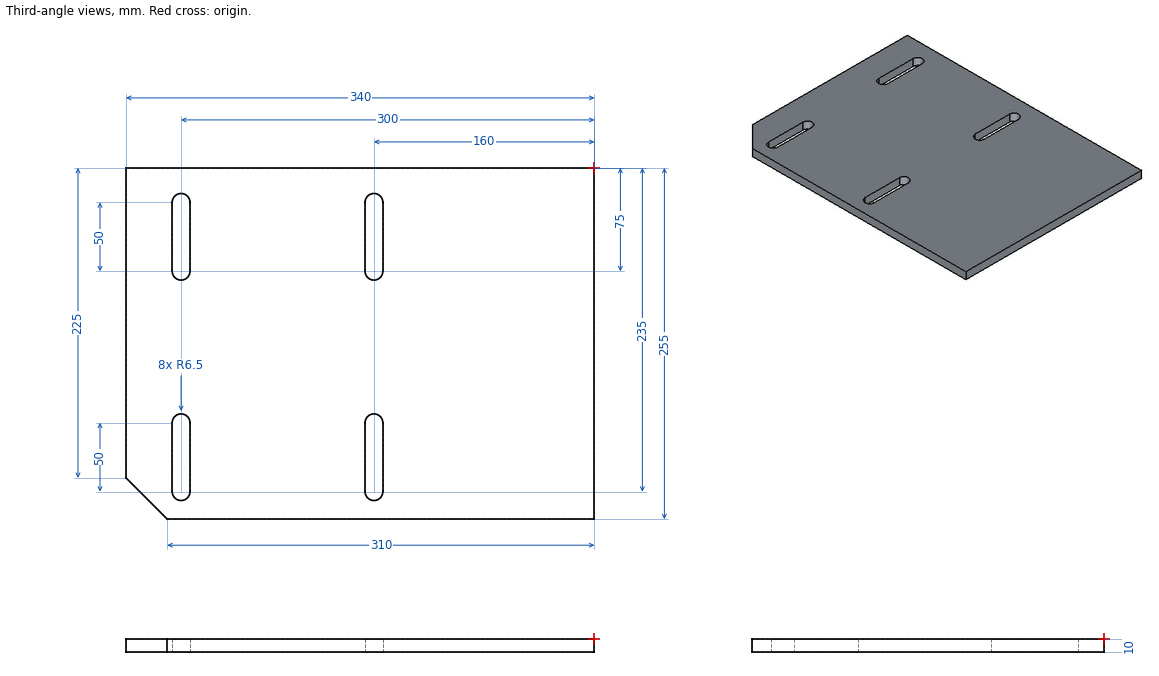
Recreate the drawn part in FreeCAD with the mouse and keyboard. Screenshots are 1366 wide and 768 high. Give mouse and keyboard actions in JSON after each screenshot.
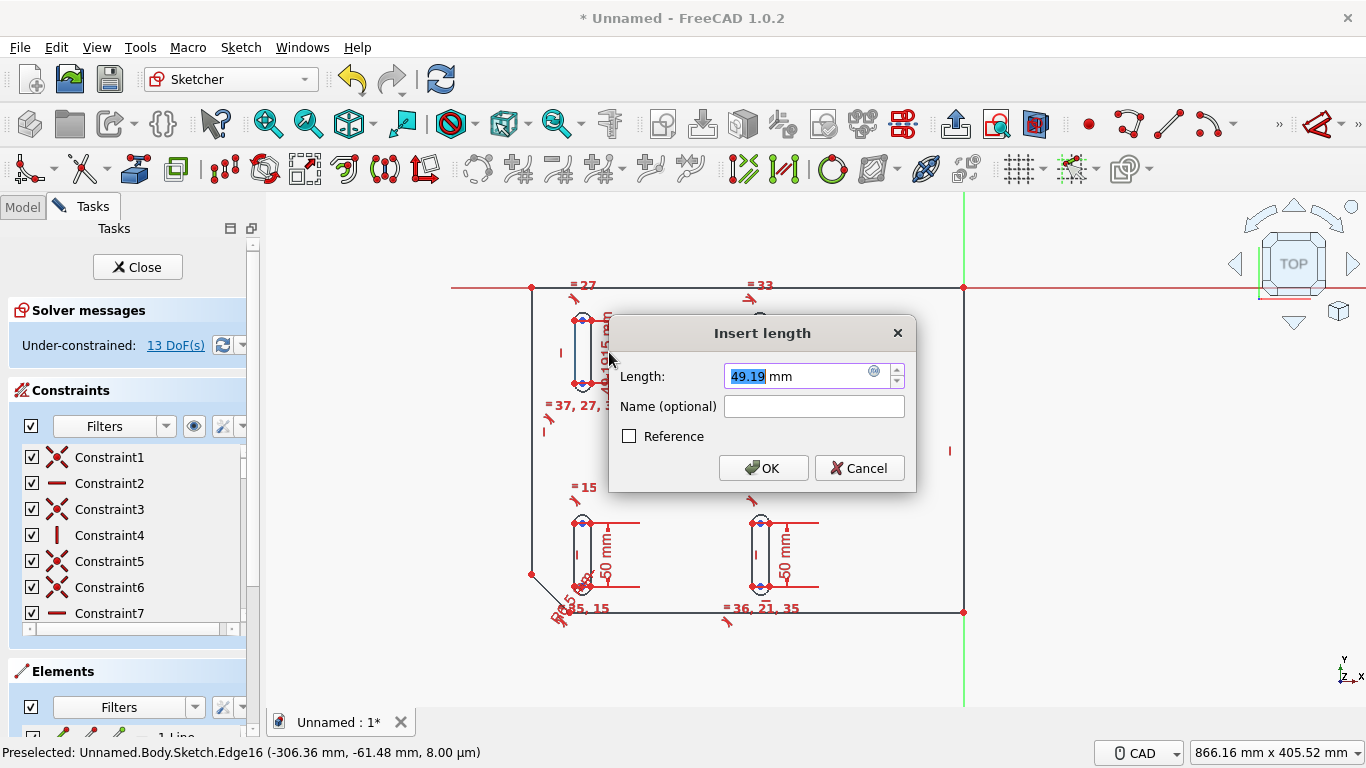
{"action": "type", "text": "50"}
{"action": "key", "text": "Return"}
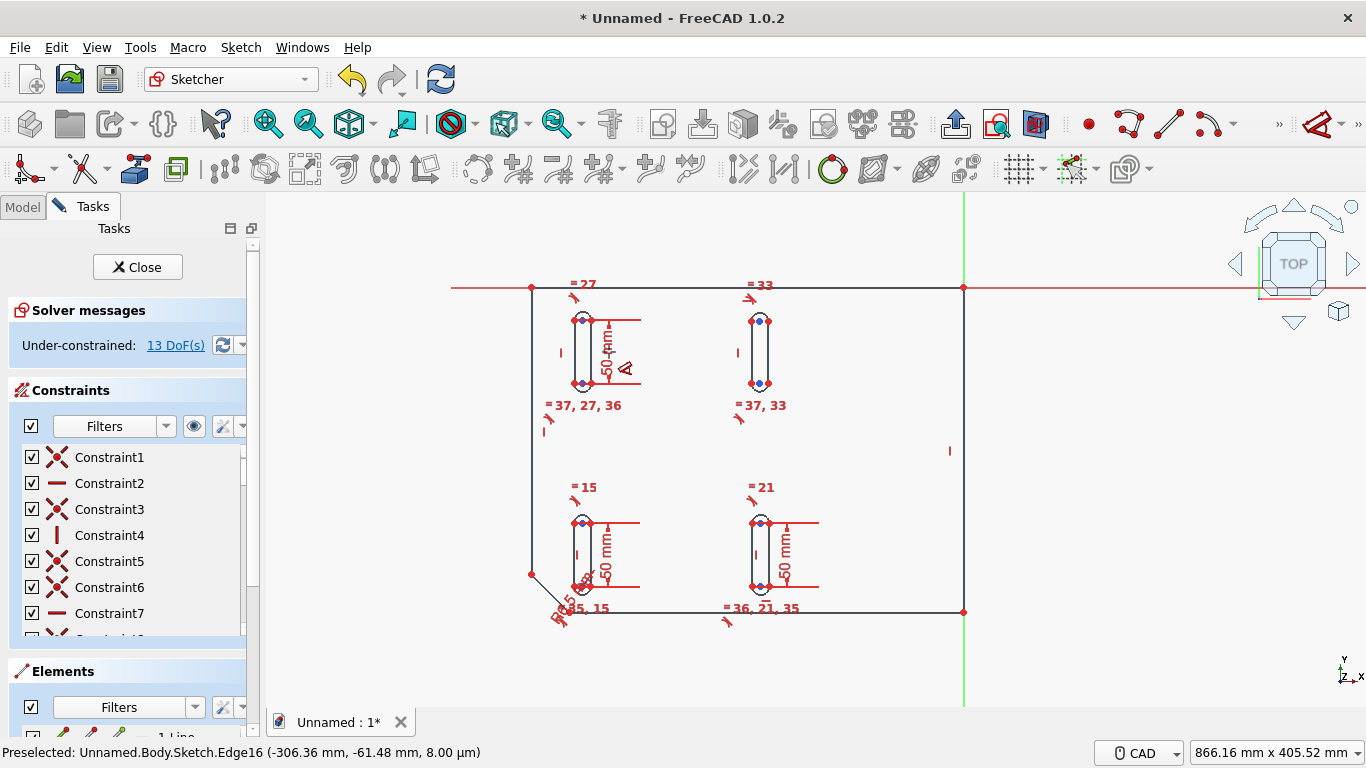
{"action": "left_click", "coordinate": [752, 365]}
{"action": "left_click", "coordinate": [786, 352]}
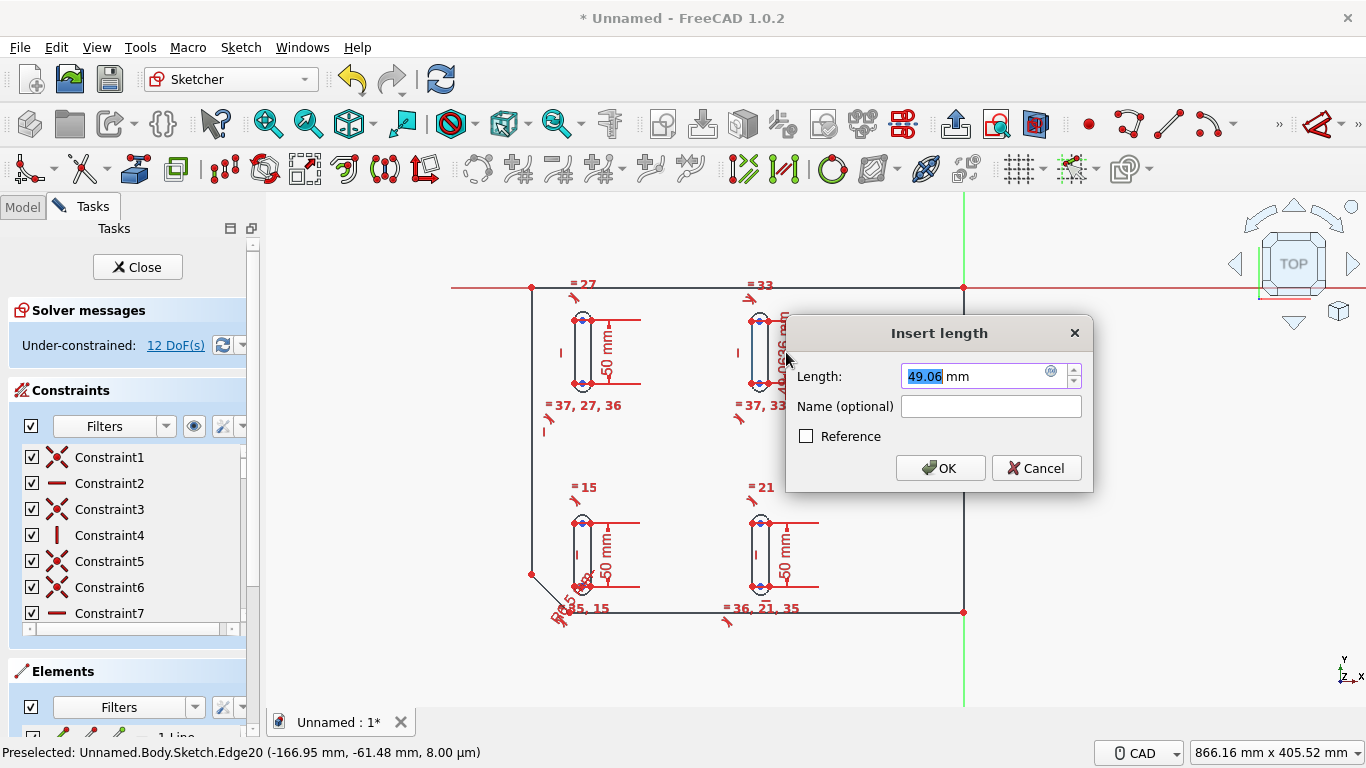
{"action": "type", "text": "50"}
{"action": "key", "text": "Return"}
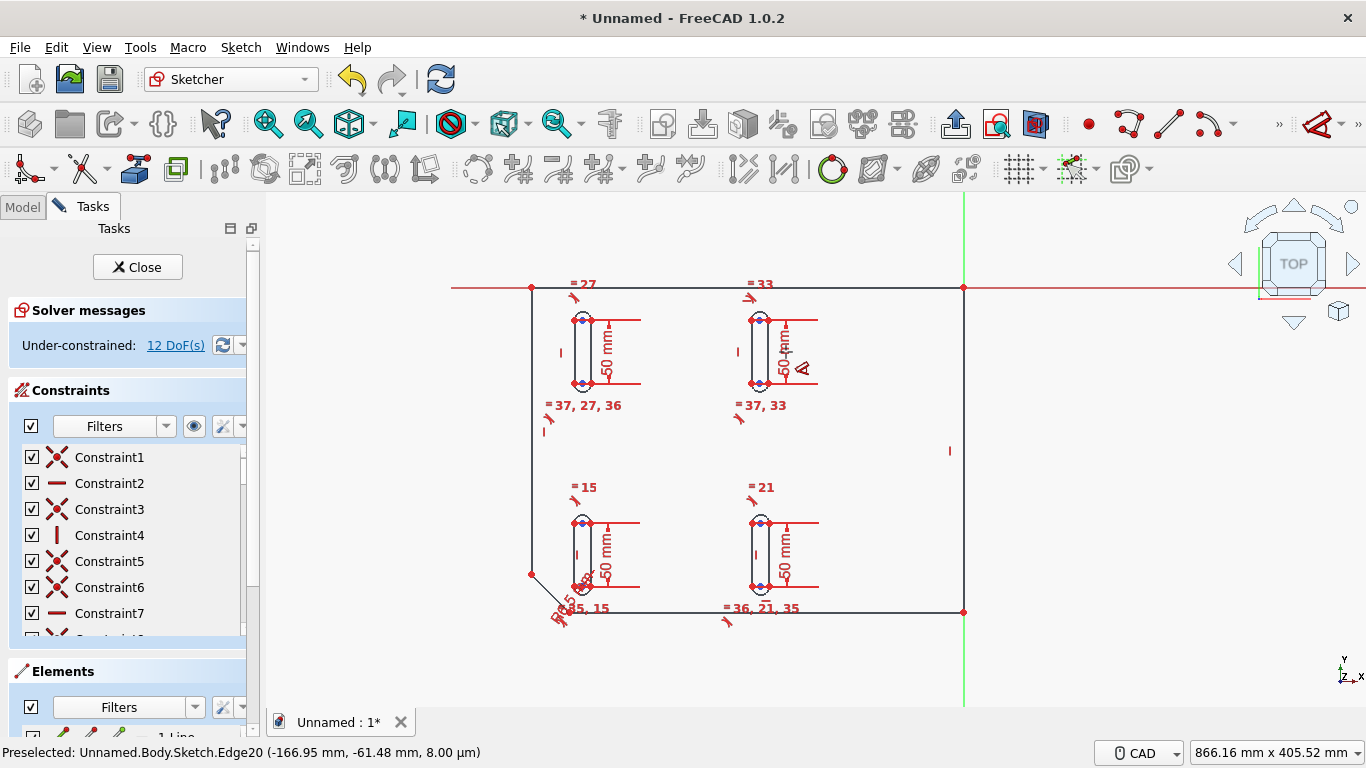
{"action": "left_click", "coordinate": [834, 288]}
{"action": "left_click", "coordinate": [748, 254]}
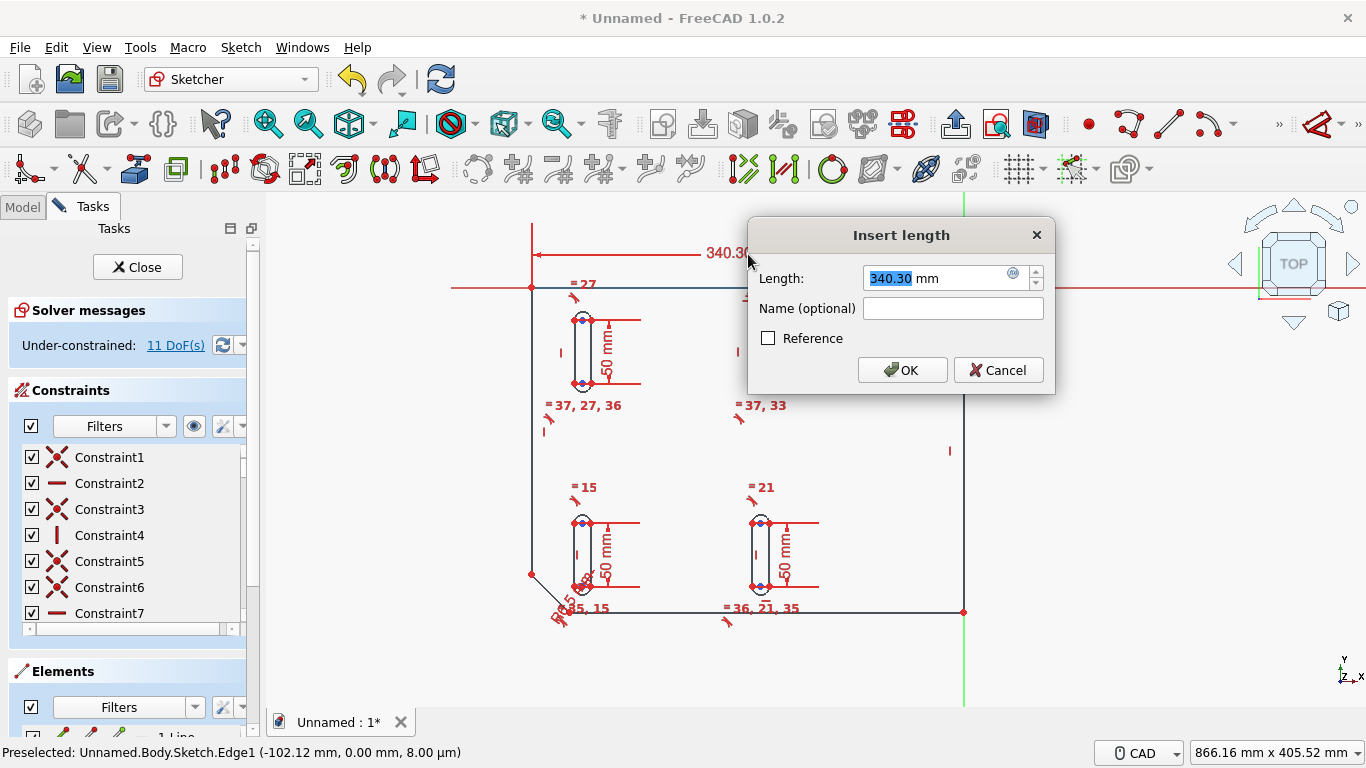
{"action": "type", "text": "340"}
{"action": "key", "text": "Return"}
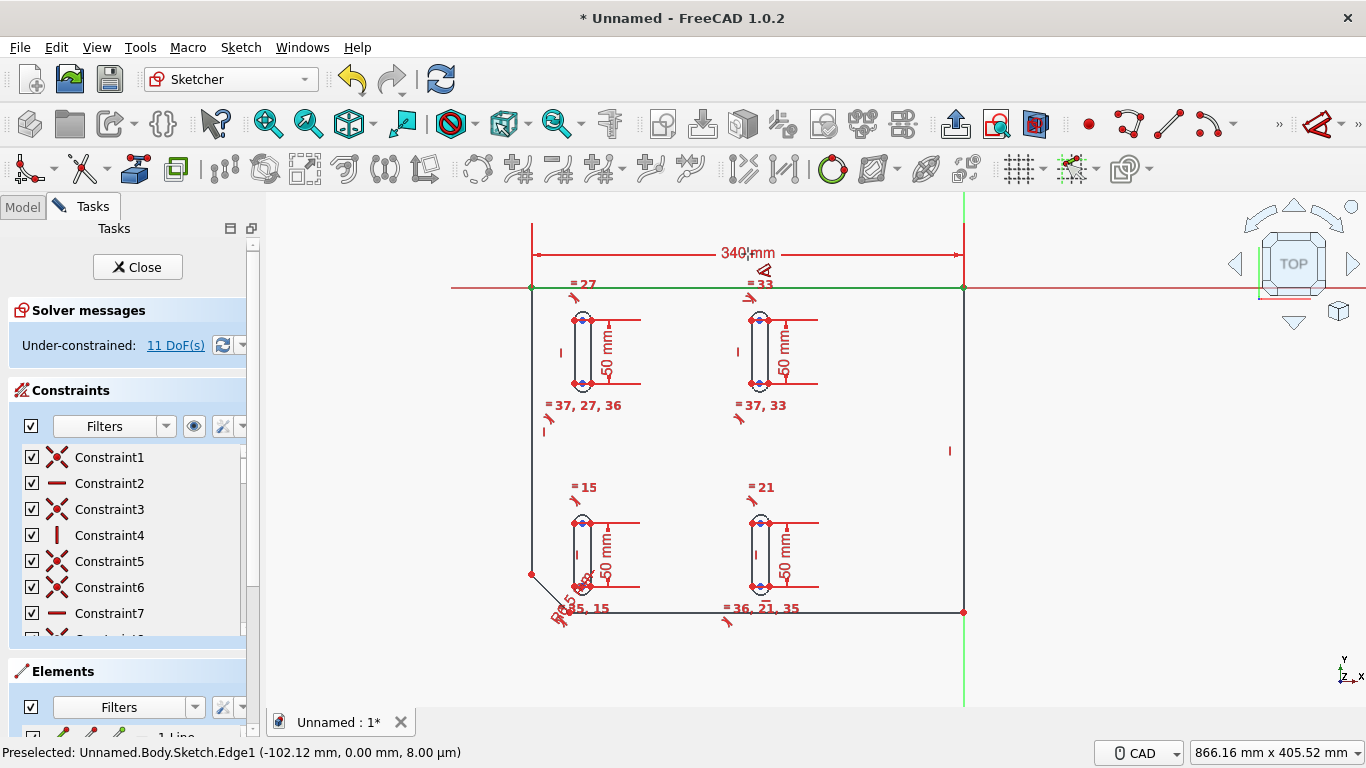
{"action": "left_click", "coordinate": [532, 374]}
{"action": "left_click", "coordinate": [498, 431]}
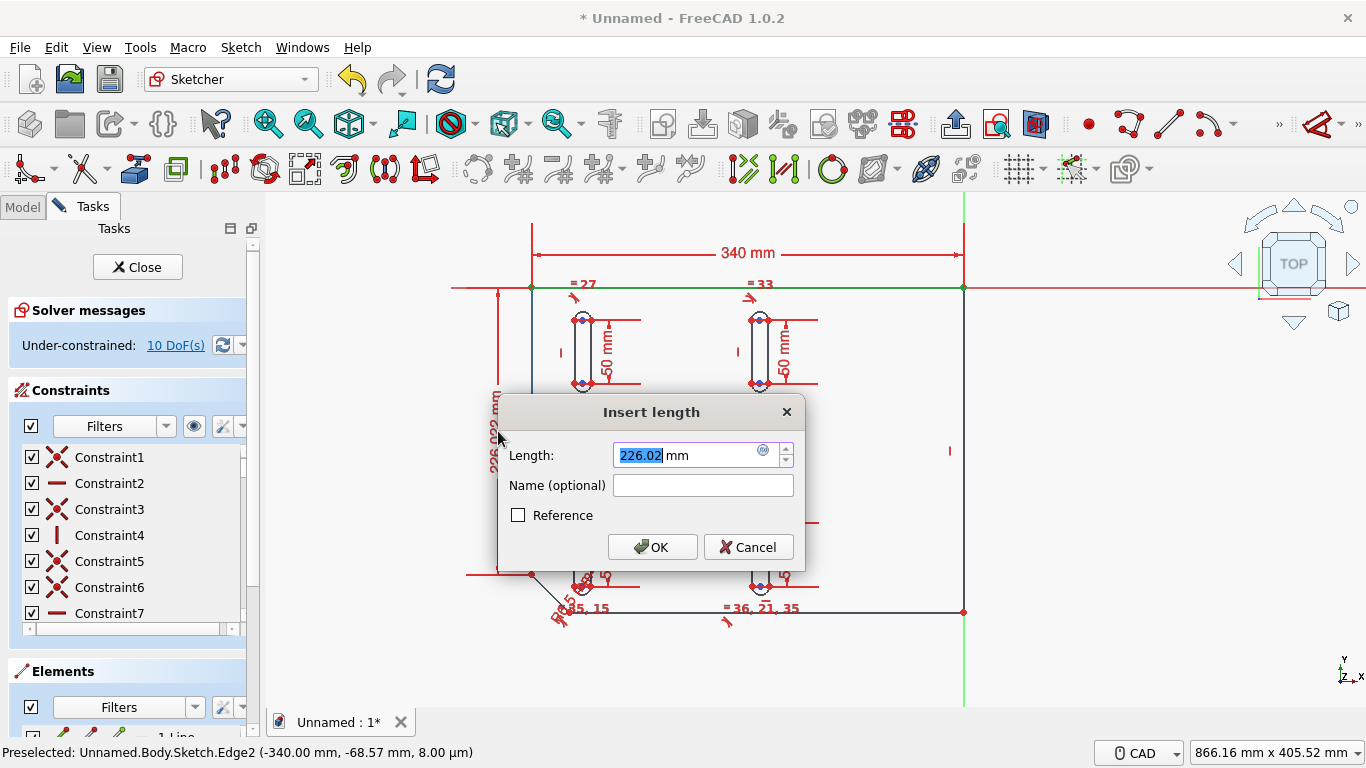
{"action": "type", "text": "225"}
{"action": "key", "text": "Return"}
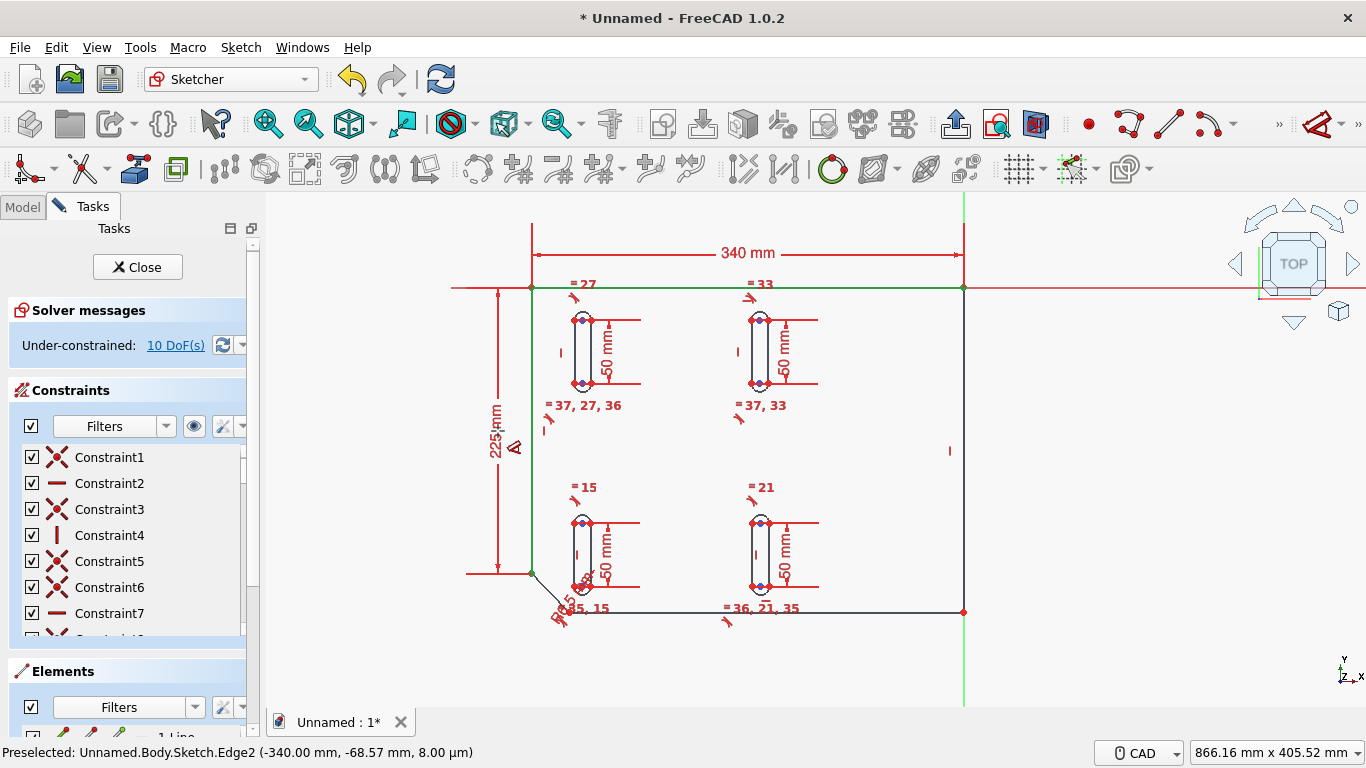
{"action": "left_click", "coordinate": [688, 613]}
{"action": "left_click", "coordinate": [767, 647]}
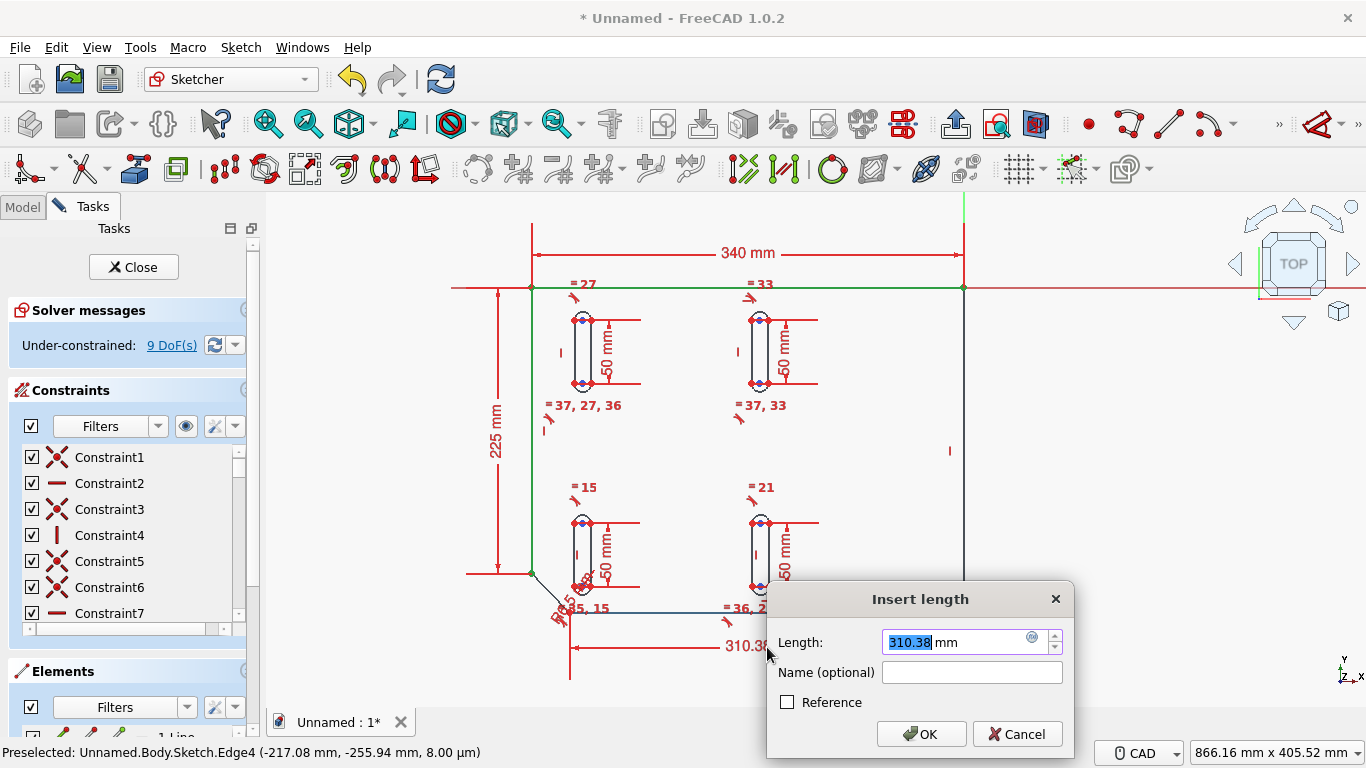
{"action": "type", "text": "310"}
{"action": "key", "text": "Return"}